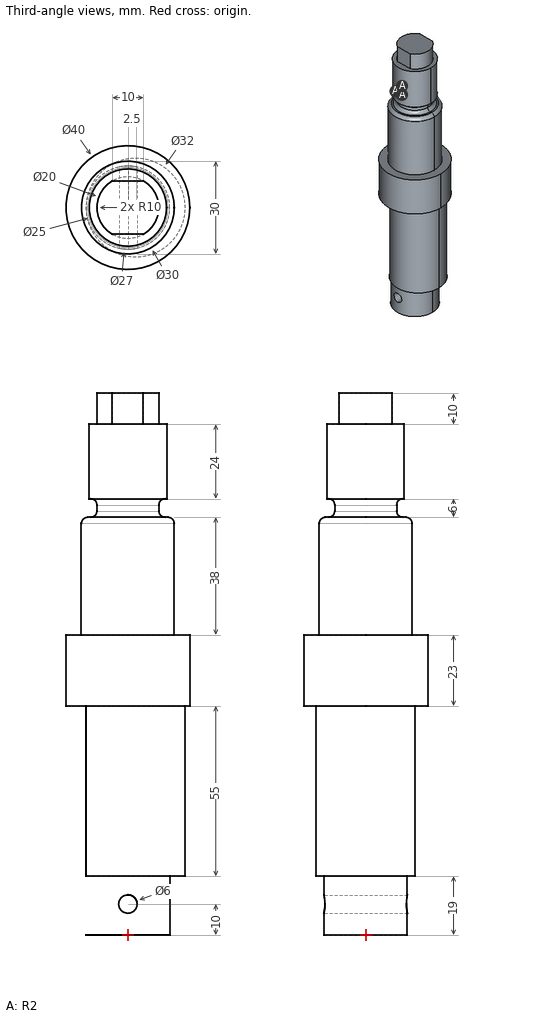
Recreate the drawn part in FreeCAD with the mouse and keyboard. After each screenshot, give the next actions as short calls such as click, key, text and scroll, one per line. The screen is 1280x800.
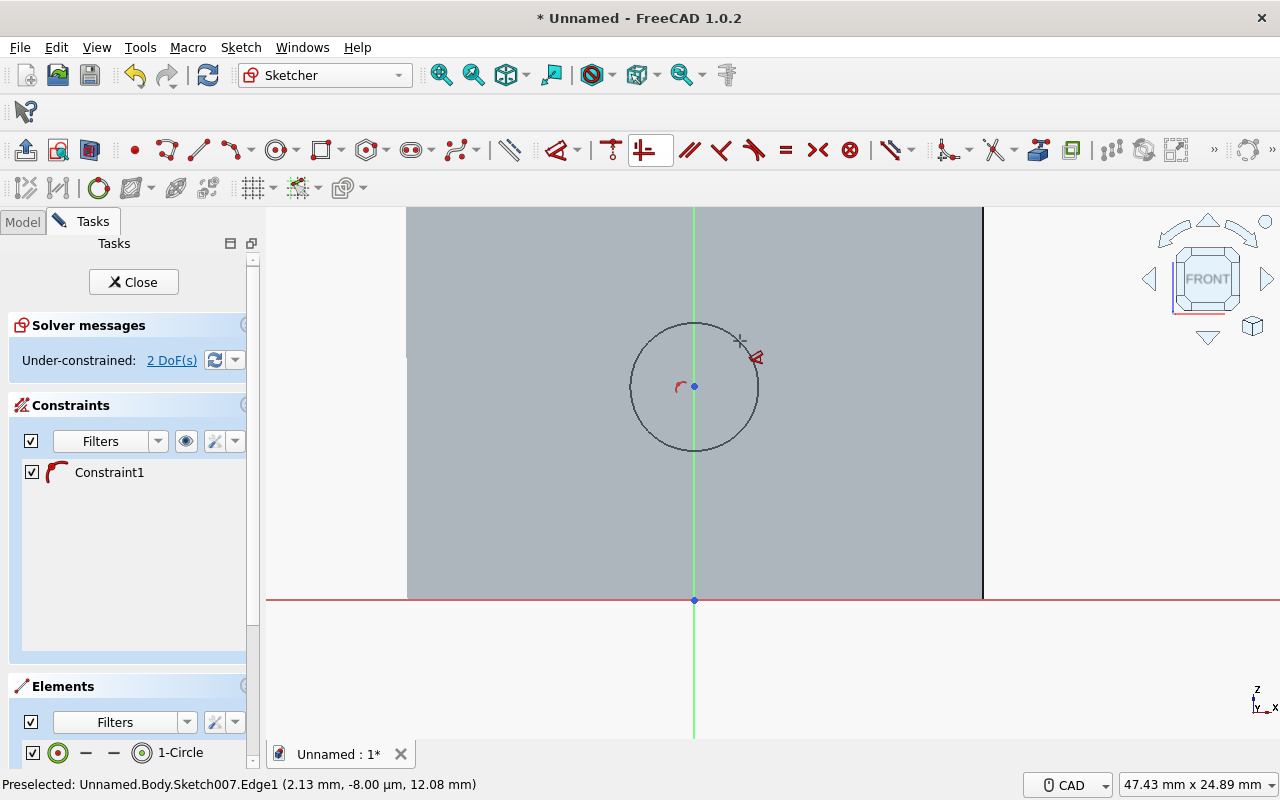
click(740, 342)
click(763, 320)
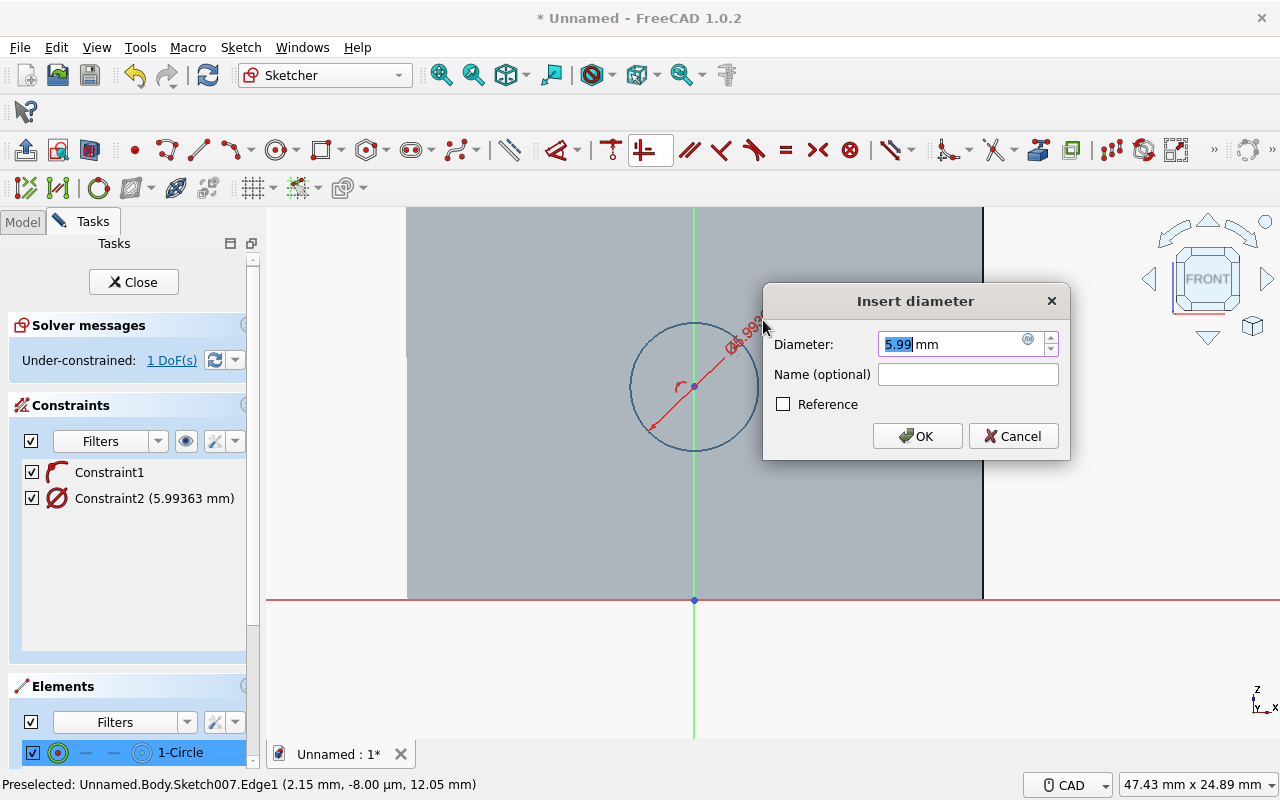
text(6)
key(Return)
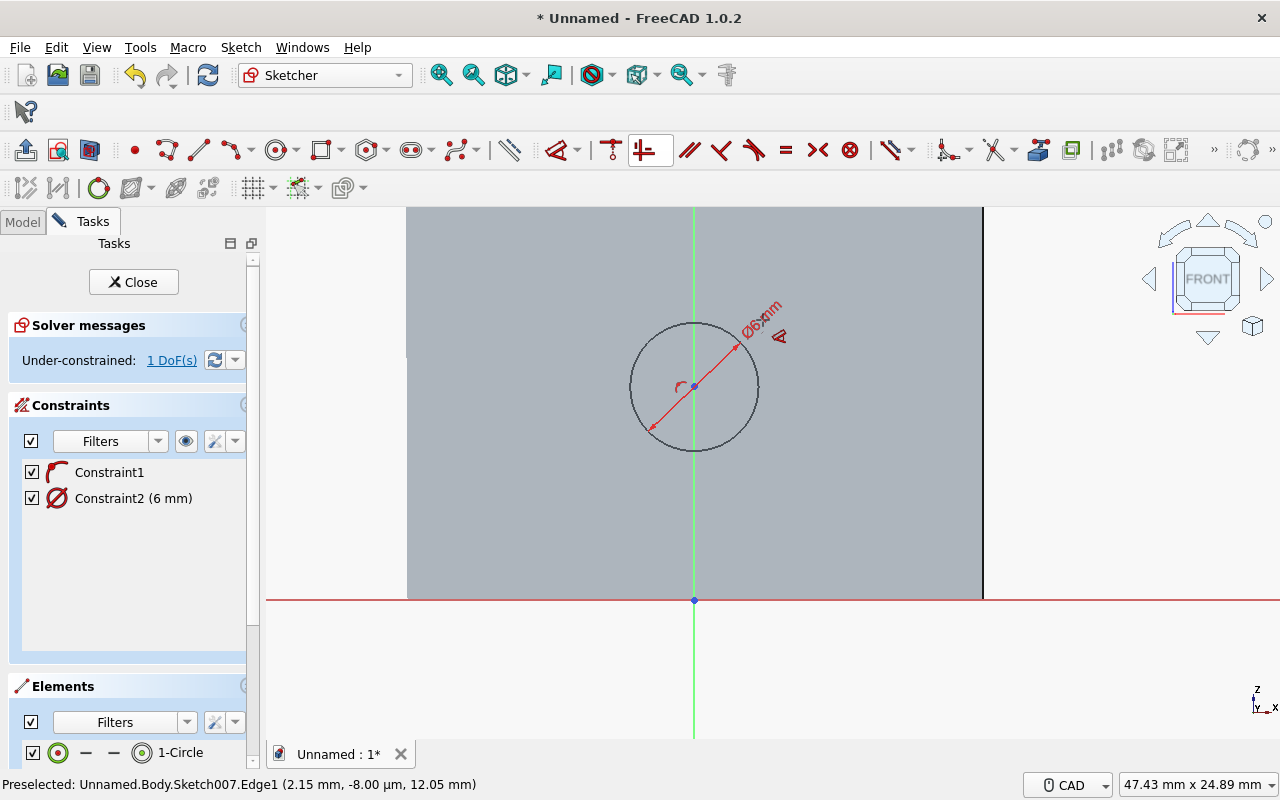
click(694, 387)
click(728, 494)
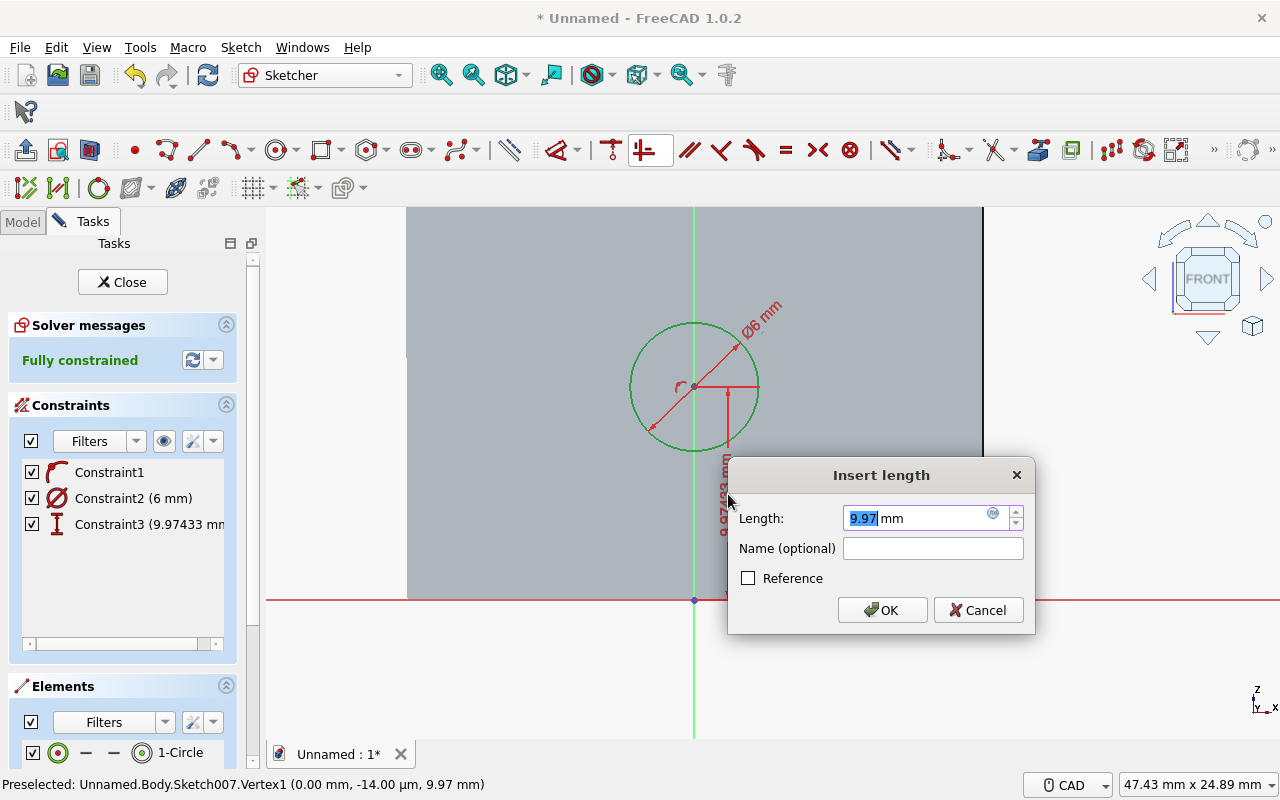
text(10)
key(Return)
key(Escape)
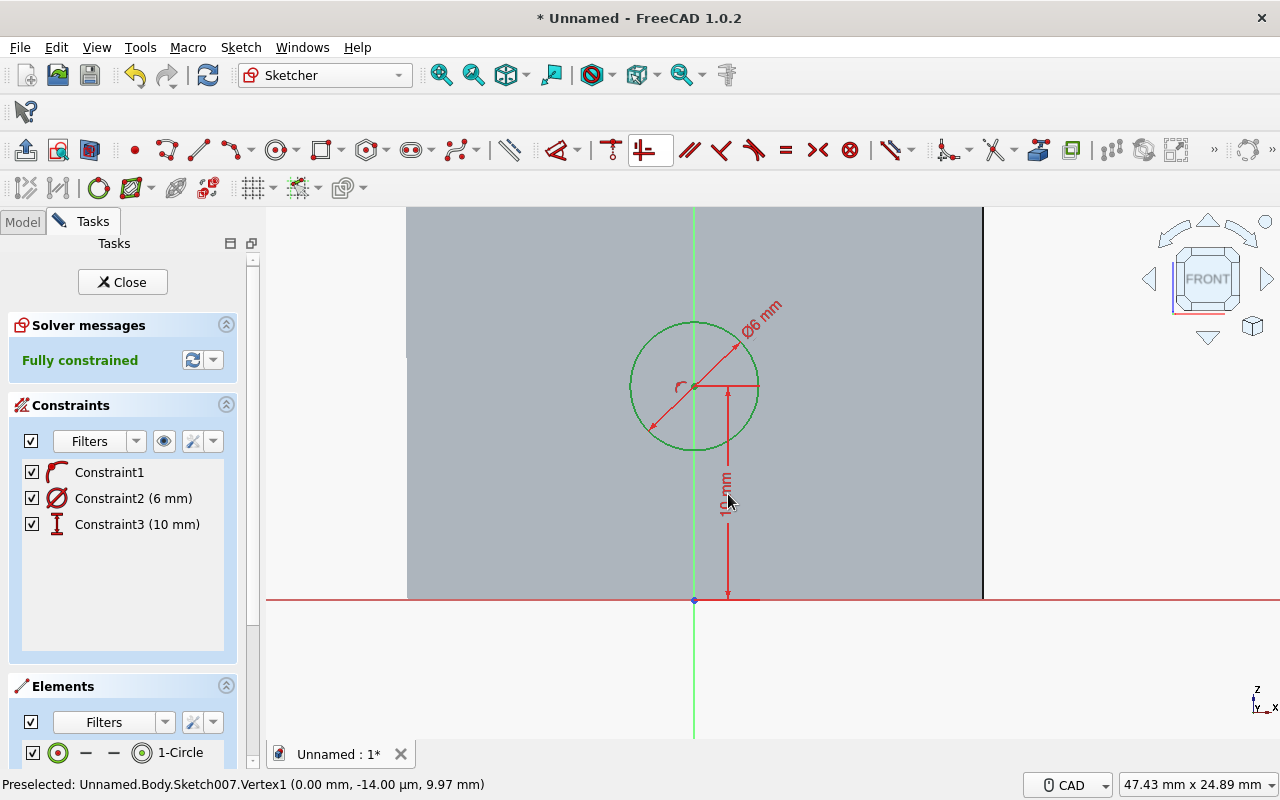
click(123, 282)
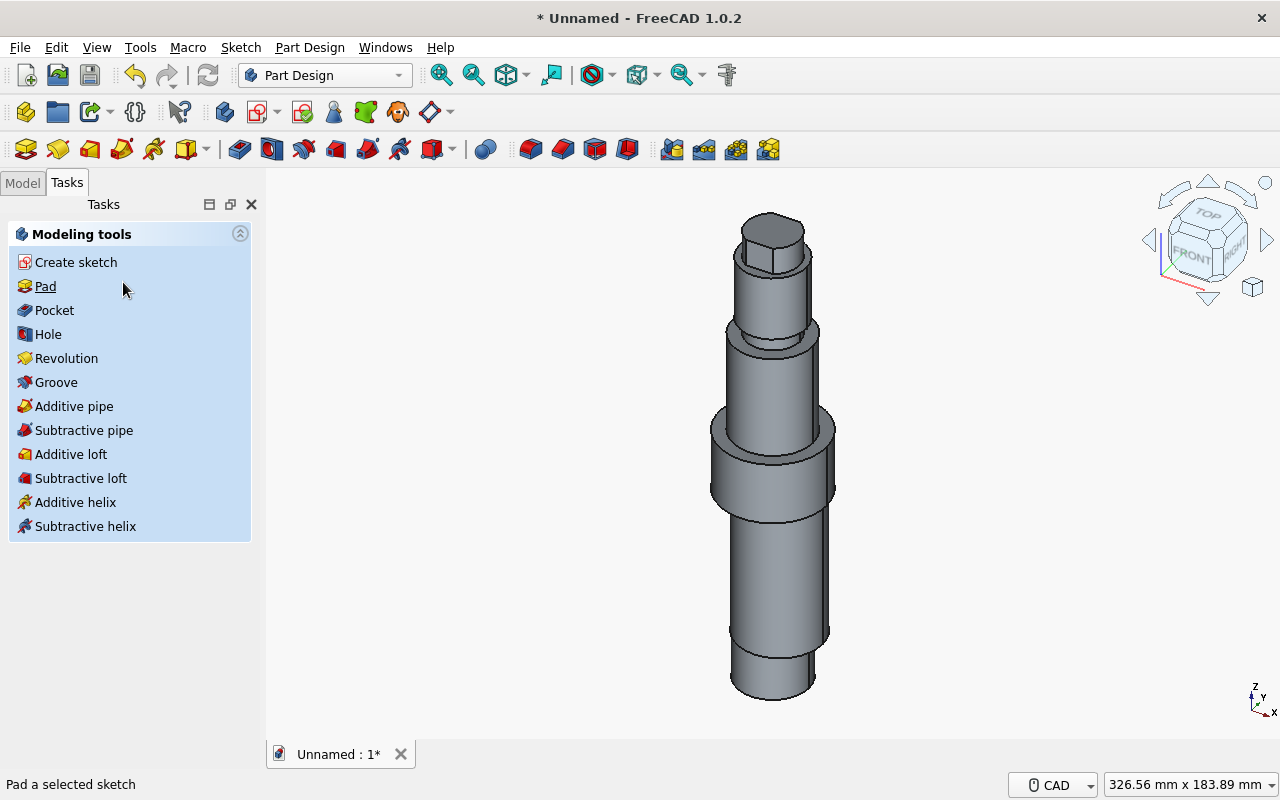
click(240, 150)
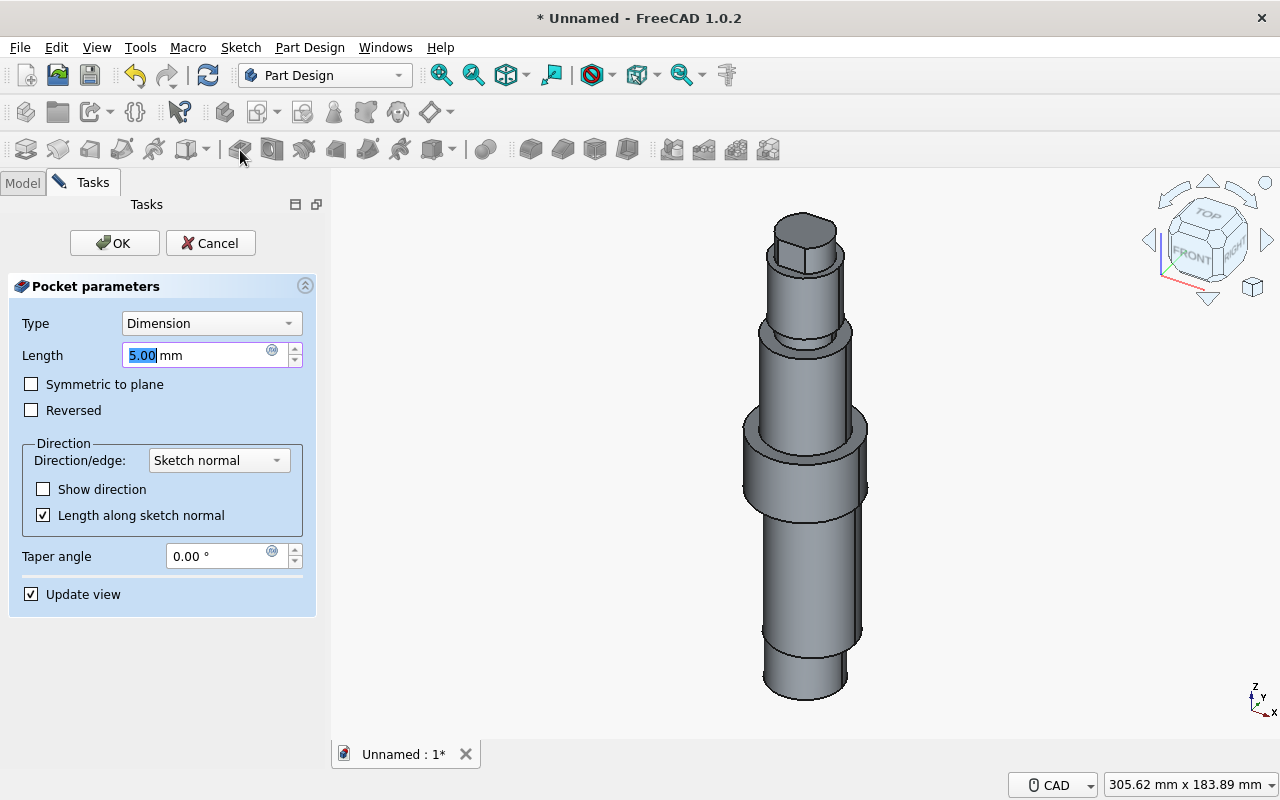
text(30)
key(Tab)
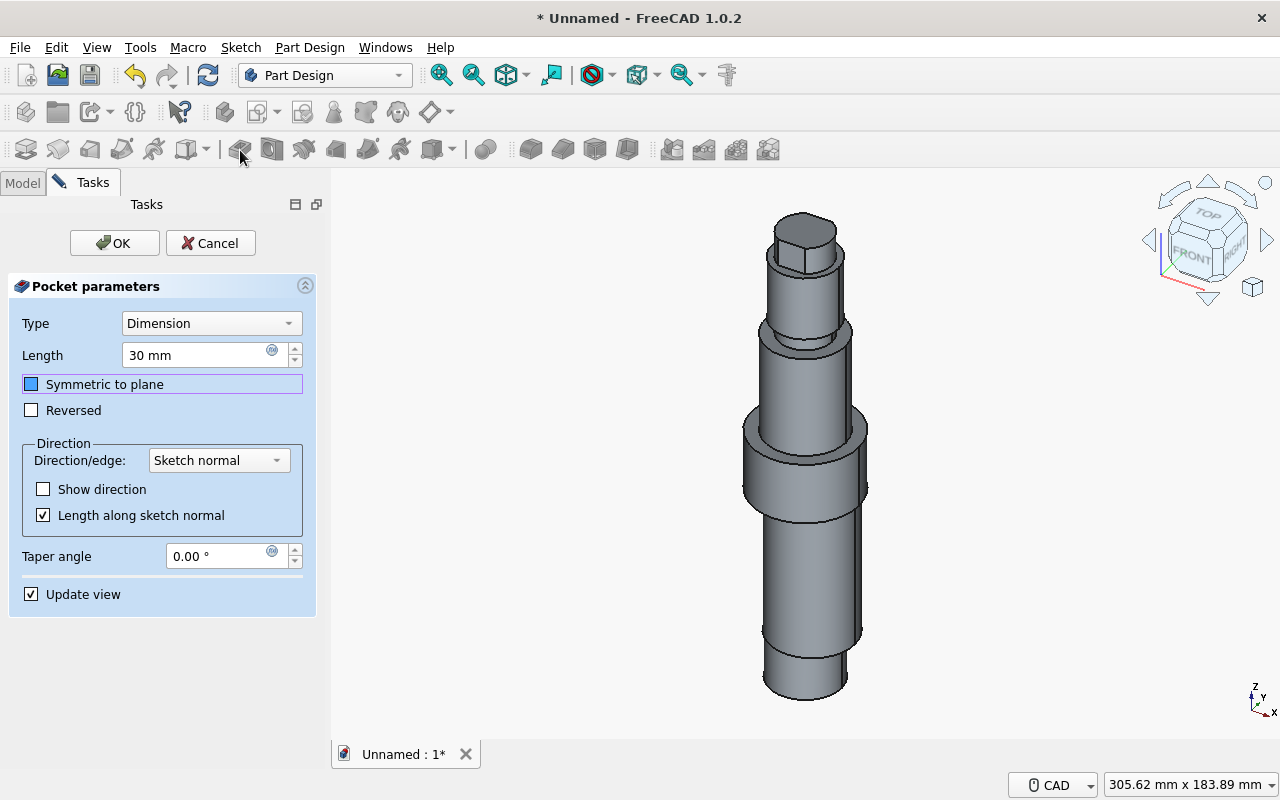
click(30, 384)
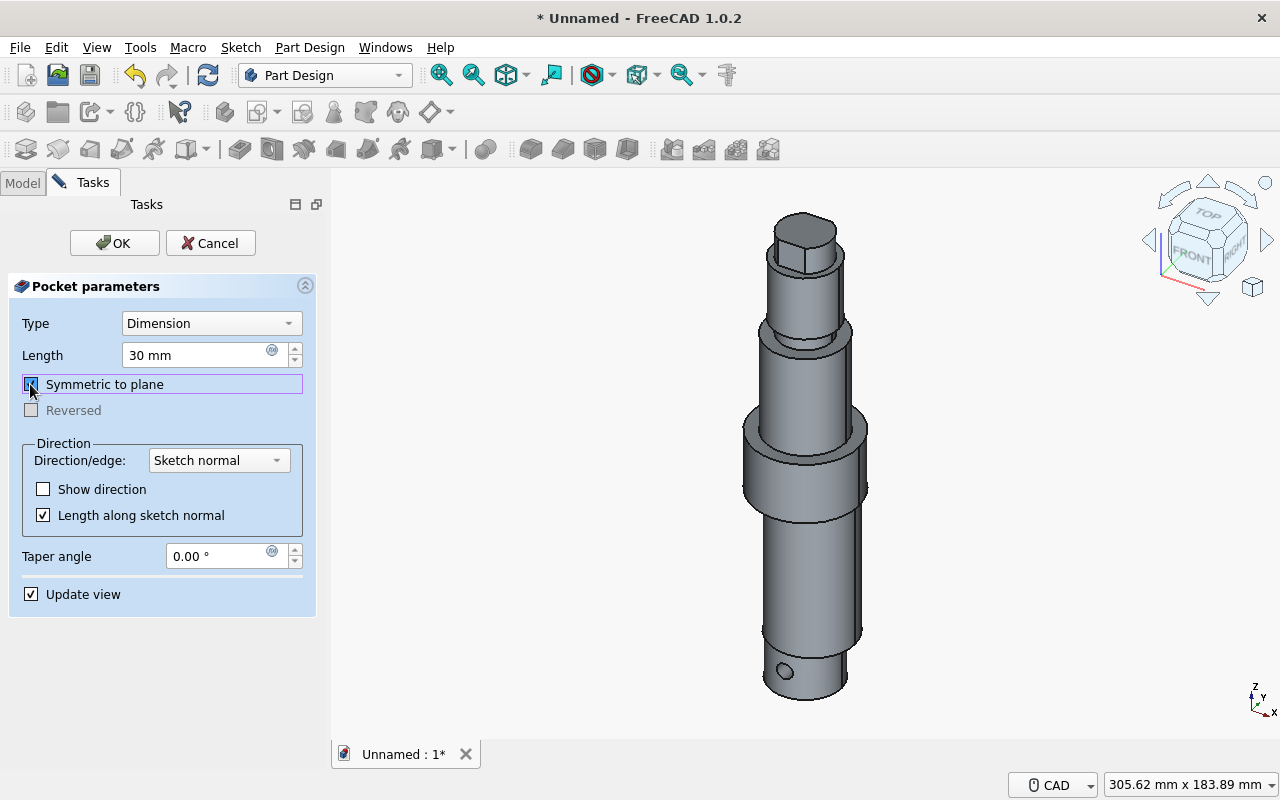
click(115, 243)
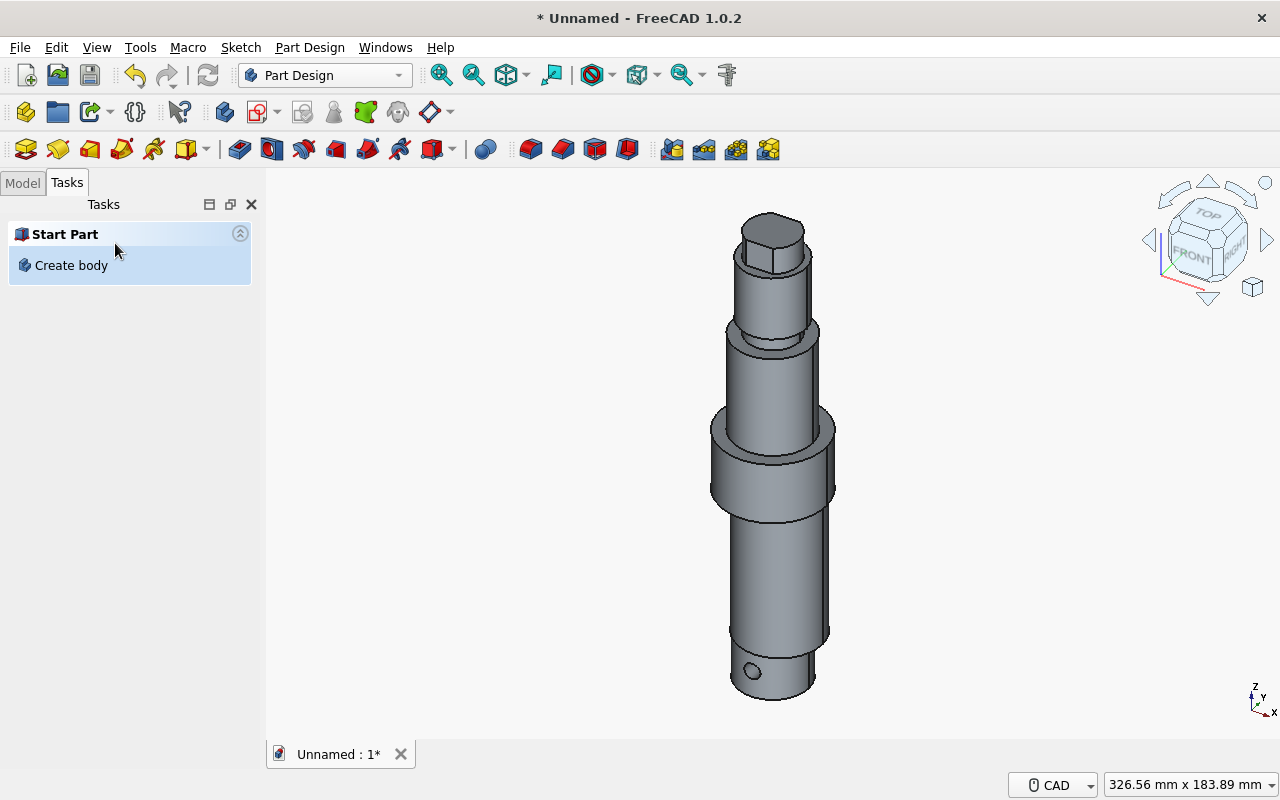
click(727, 334)